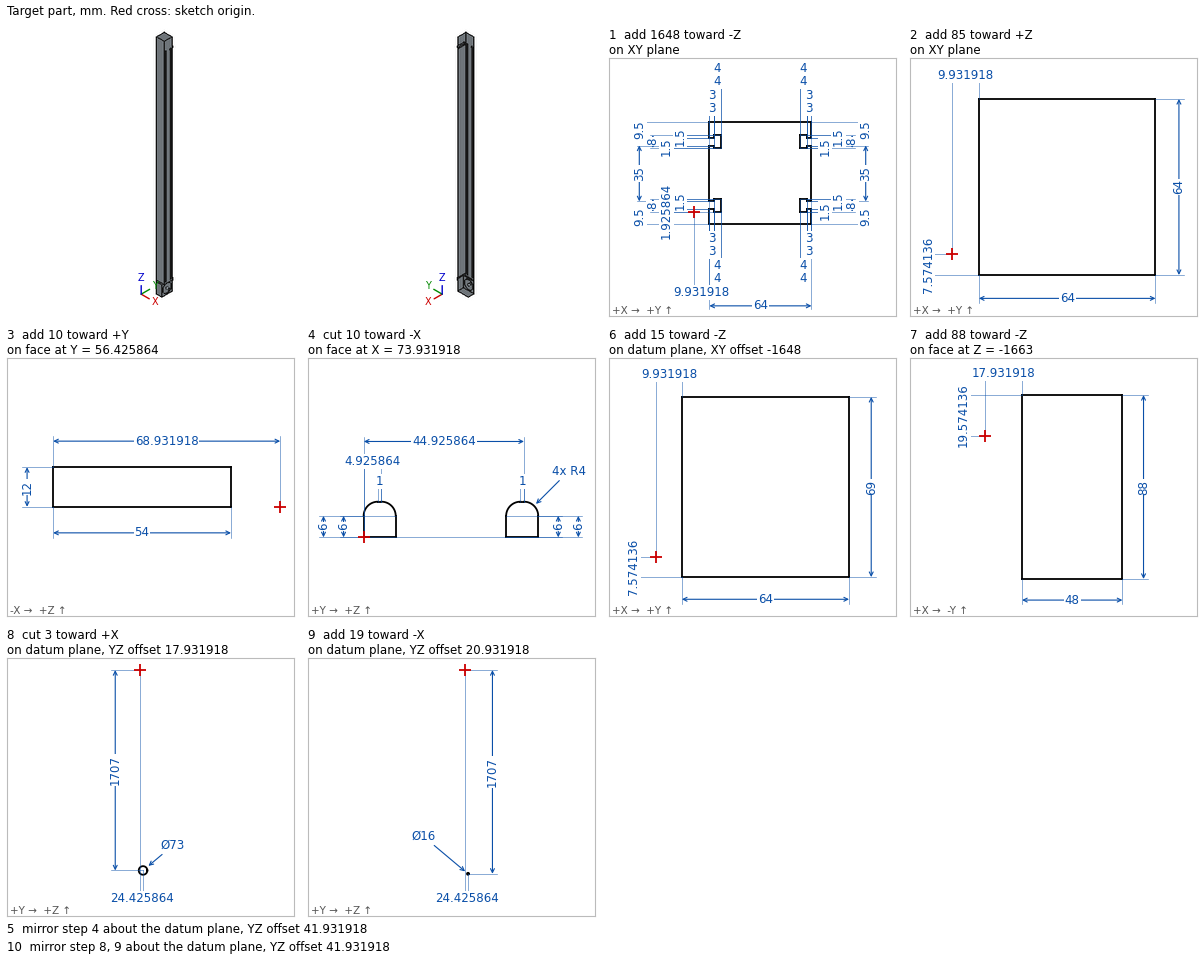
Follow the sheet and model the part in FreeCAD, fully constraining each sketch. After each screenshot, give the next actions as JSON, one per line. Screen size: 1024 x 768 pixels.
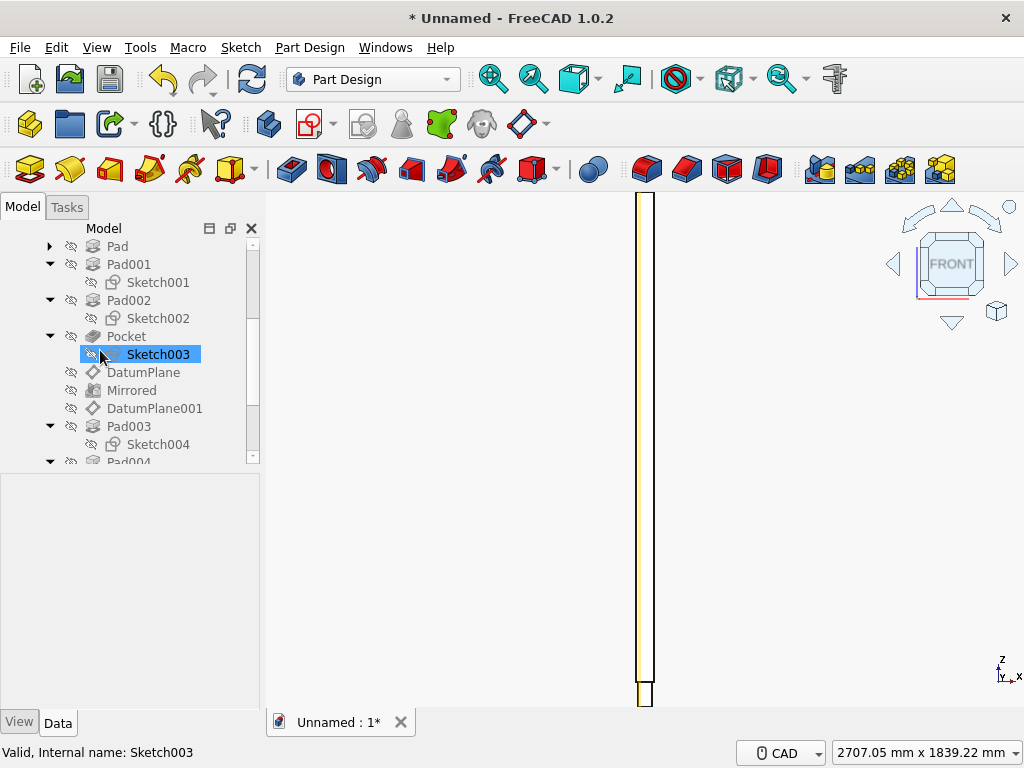
{"action": "scroll", "coordinate": [140, 350], "scroll_direction": "up", "scroll_amount": 15}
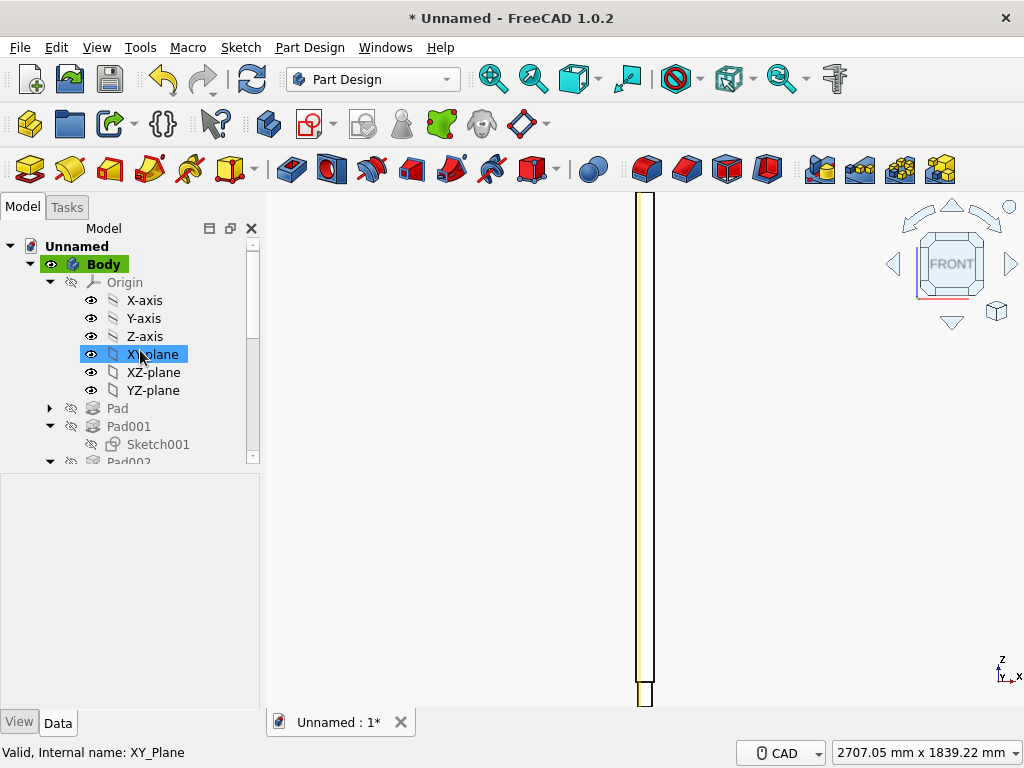
{"action": "scroll", "coordinate": [100, 350], "scroll_direction": "down", "scroll_amount": 6}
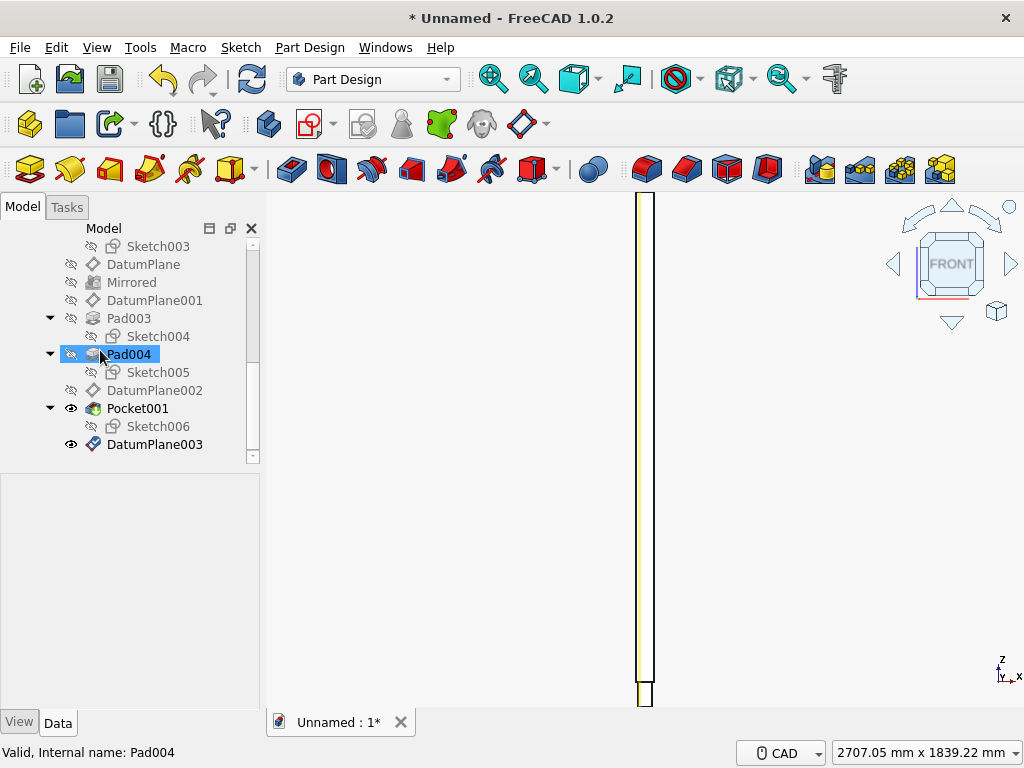
{"action": "left_click", "coordinate": [116, 444]}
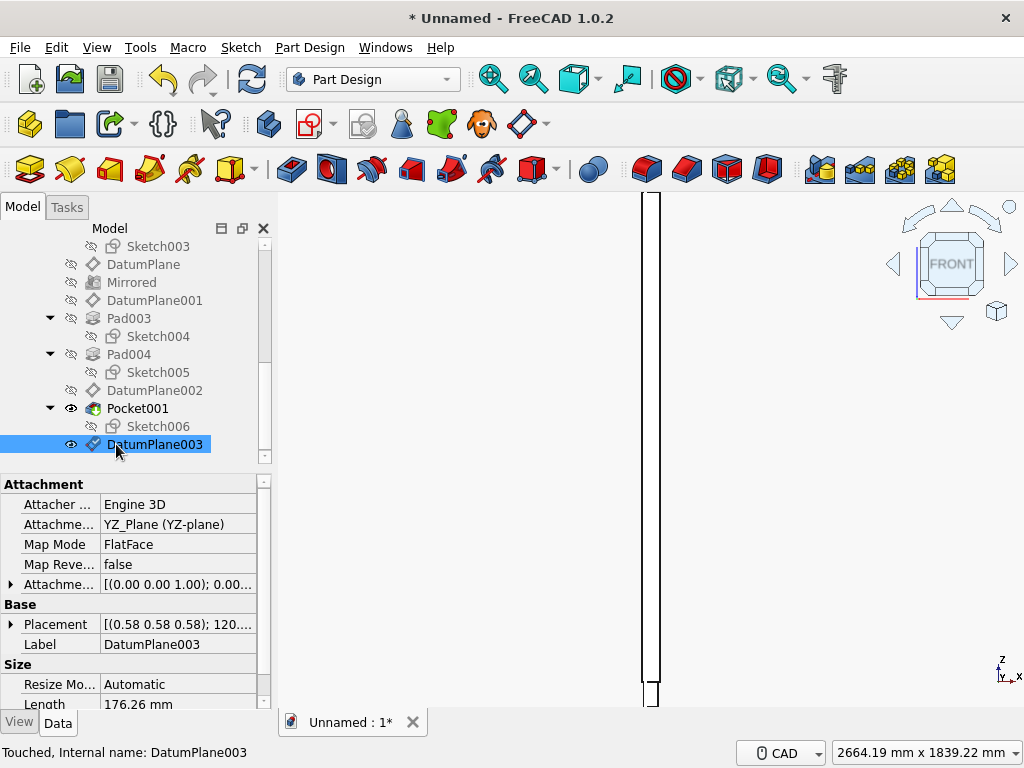
{"action": "left_click", "coordinate": [310, 124]}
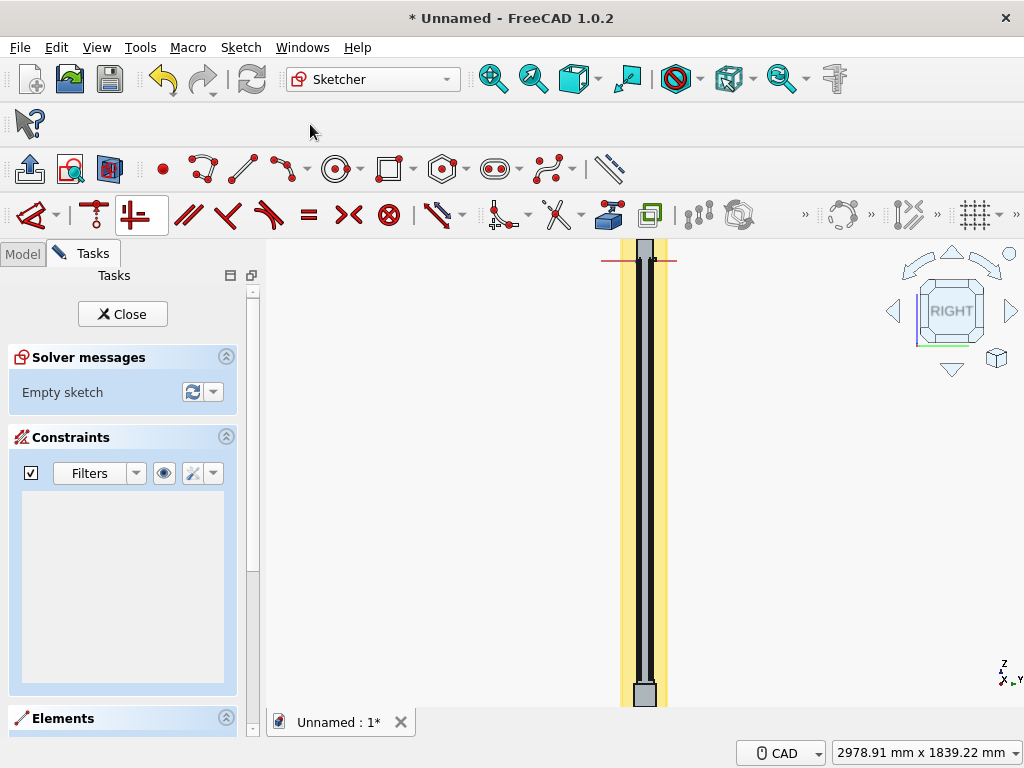
{"action": "left_click", "coordinate": [110, 170]}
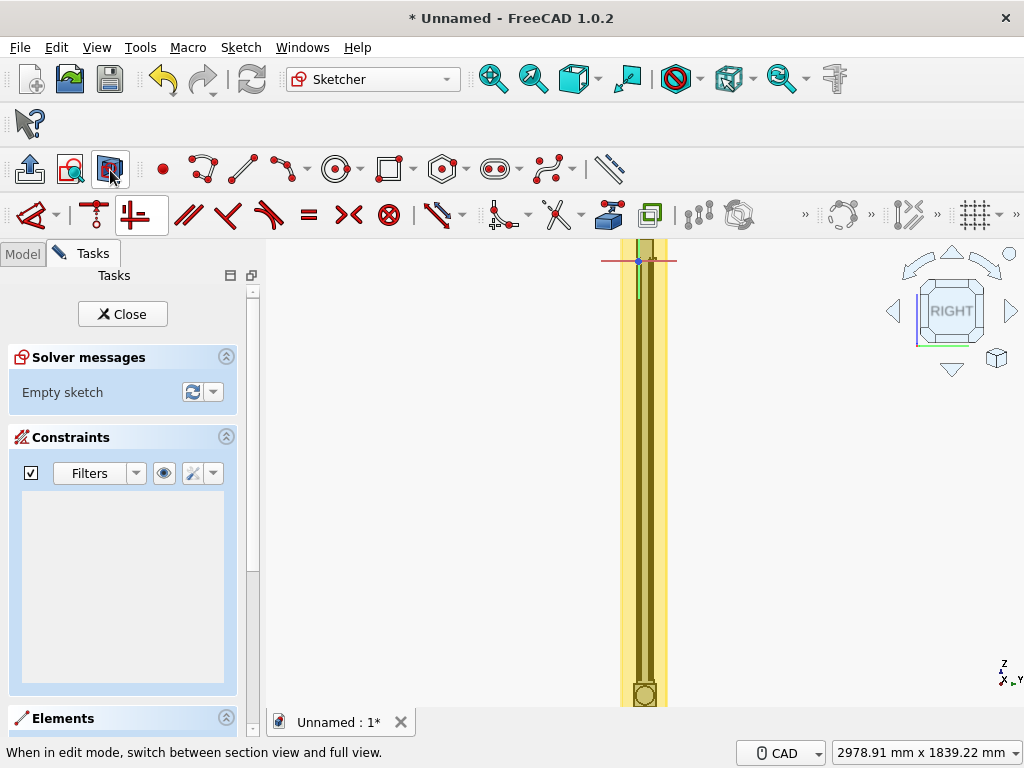
{"action": "scroll", "coordinate": [576, 473], "scroll_direction": "down", "scroll_amount": 5}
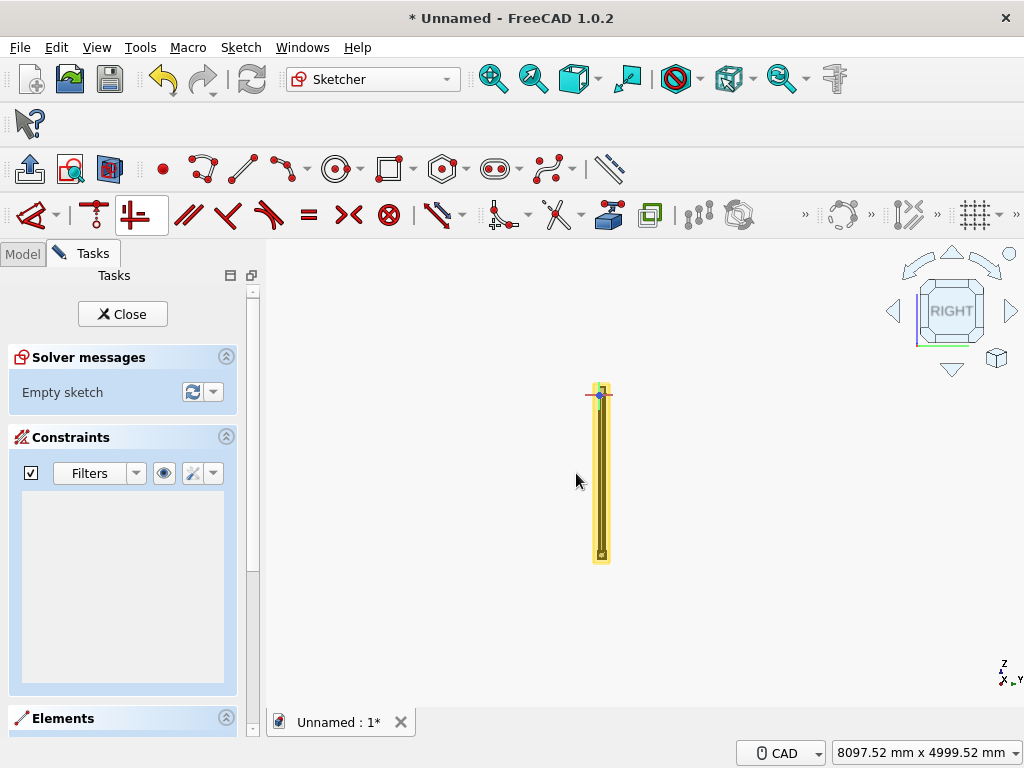
{"action": "scroll", "coordinate": [603, 559], "scroll_direction": "up", "scroll_amount": 15}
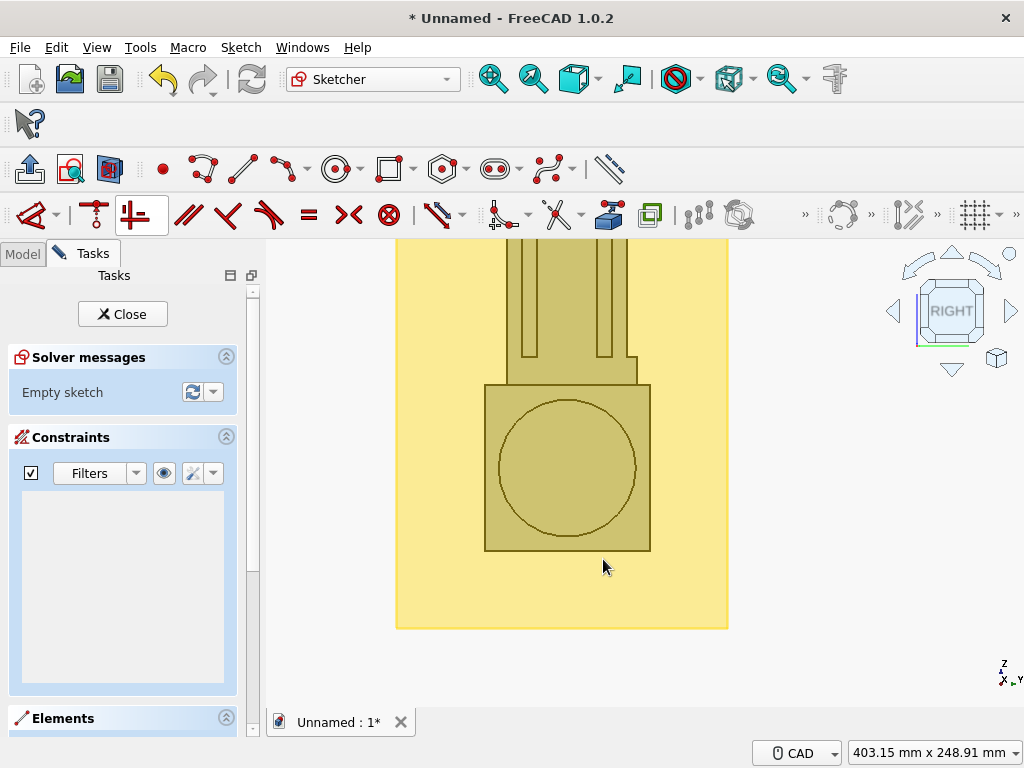
{"action": "scroll", "coordinate": [566, 468], "scroll_direction": "up", "scroll_amount": 11}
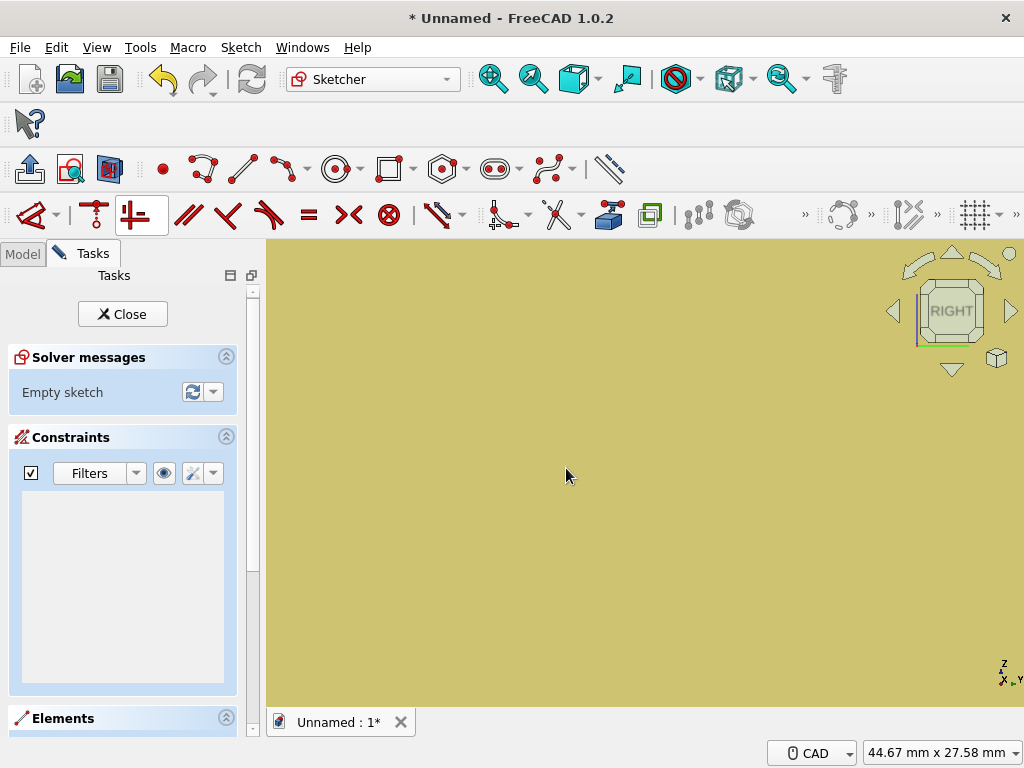
{"action": "left_click", "coordinate": [336, 170]}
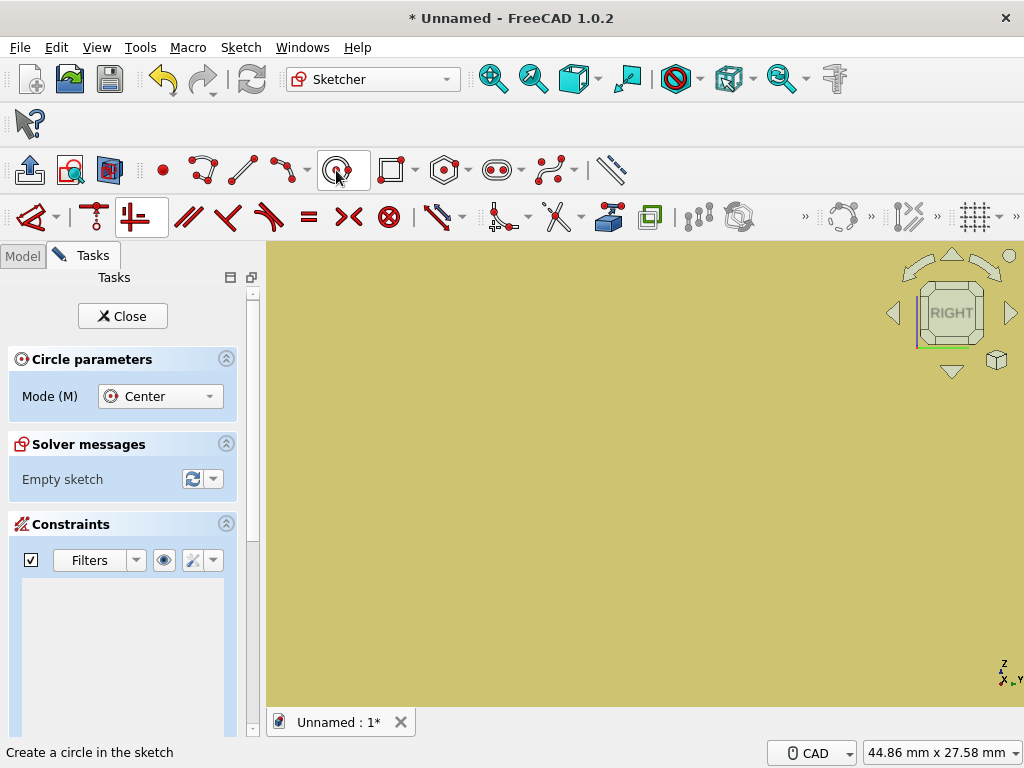
{"action": "left_click", "coordinate": [574, 467]}
{"action": "mouse_move", "coordinate": [670, 371]}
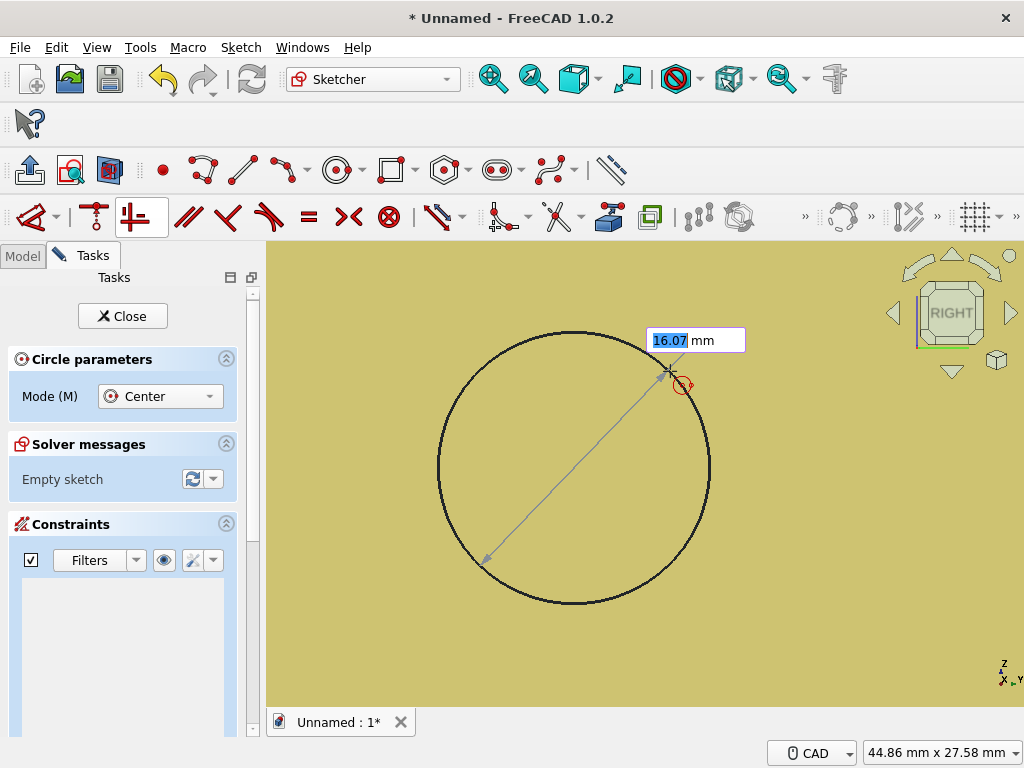
{"action": "type", "text": "16"}
{"action": "key", "text": "Return"}
{"action": "key", "text": "Escape"}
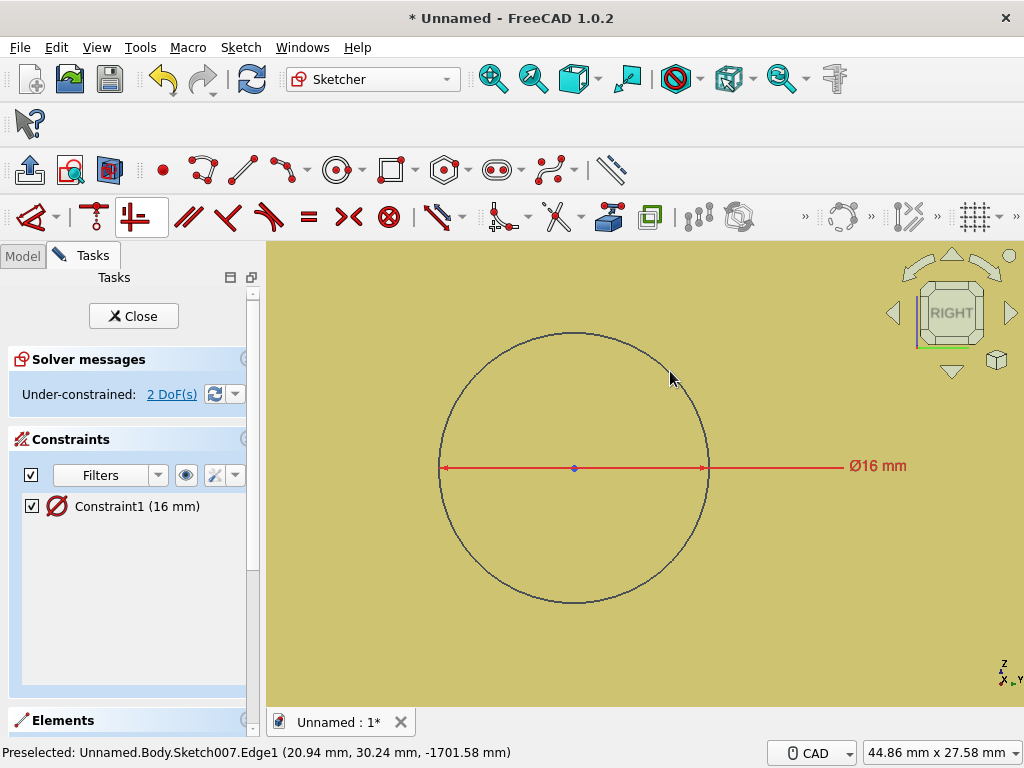
{"action": "left_click", "coordinate": [32, 218]}